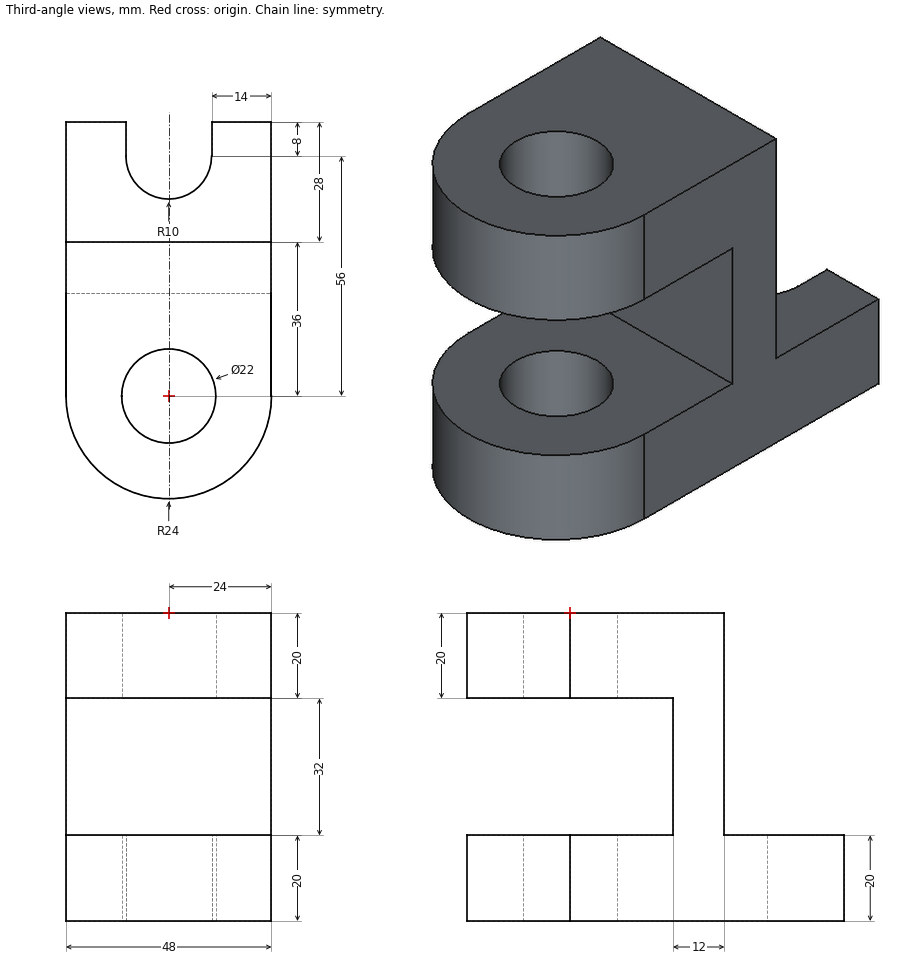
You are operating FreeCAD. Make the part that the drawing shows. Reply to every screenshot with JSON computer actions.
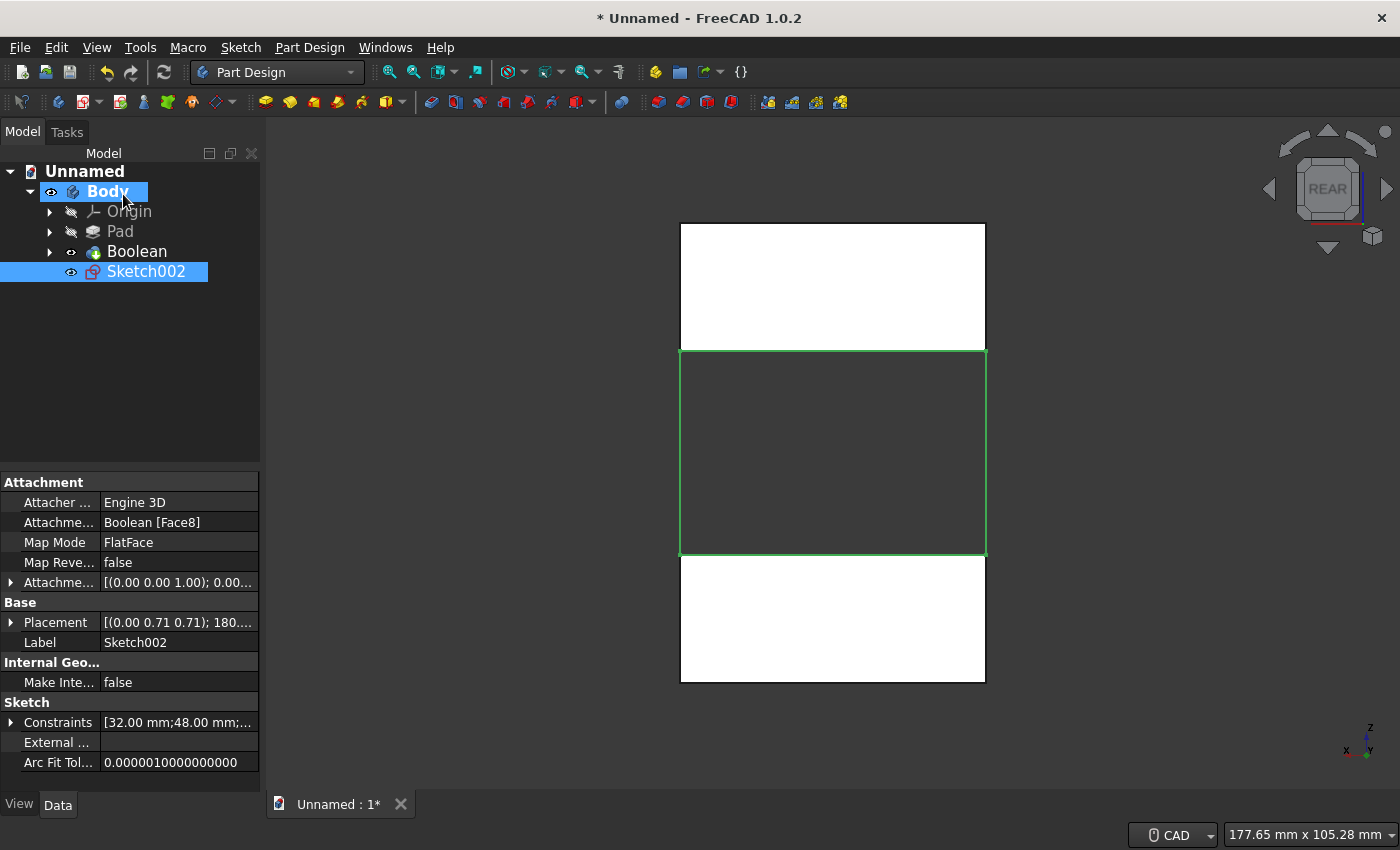
{"action": "left_click", "coordinate": [266, 102]}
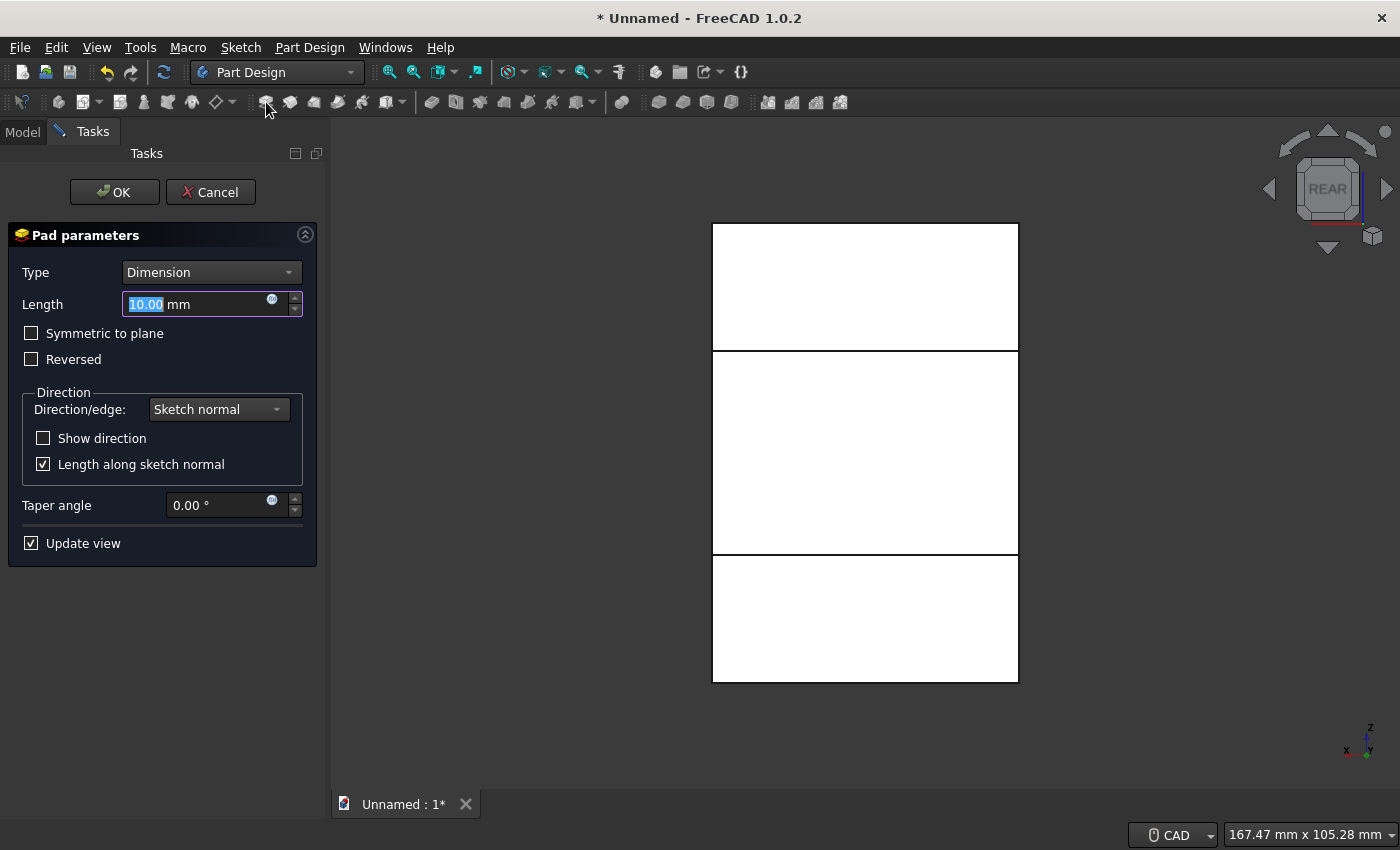
{"action": "type", "text": "12"}
{"action": "key", "text": "Tab"}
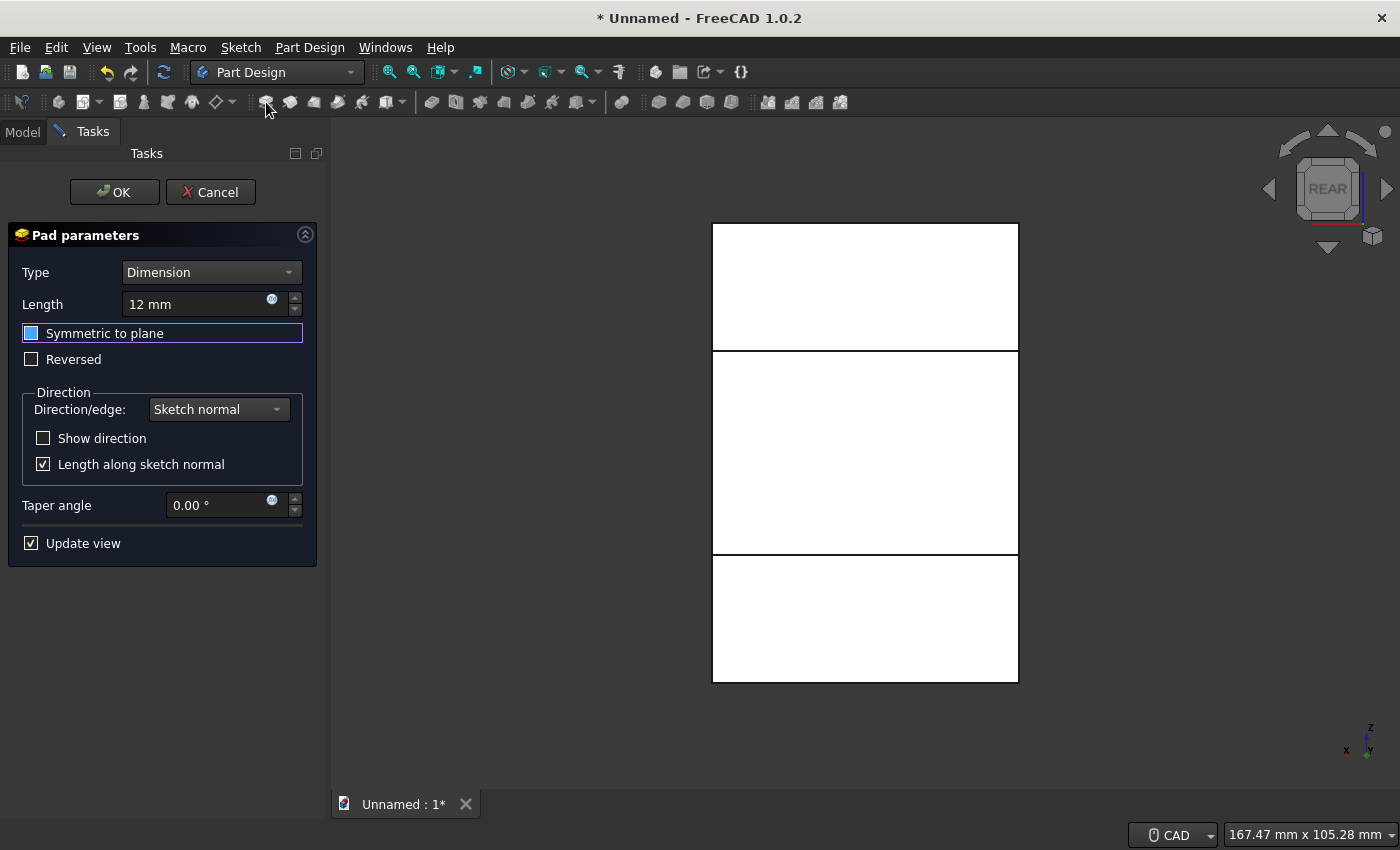
{"action": "left_click", "coordinate": [30, 359]}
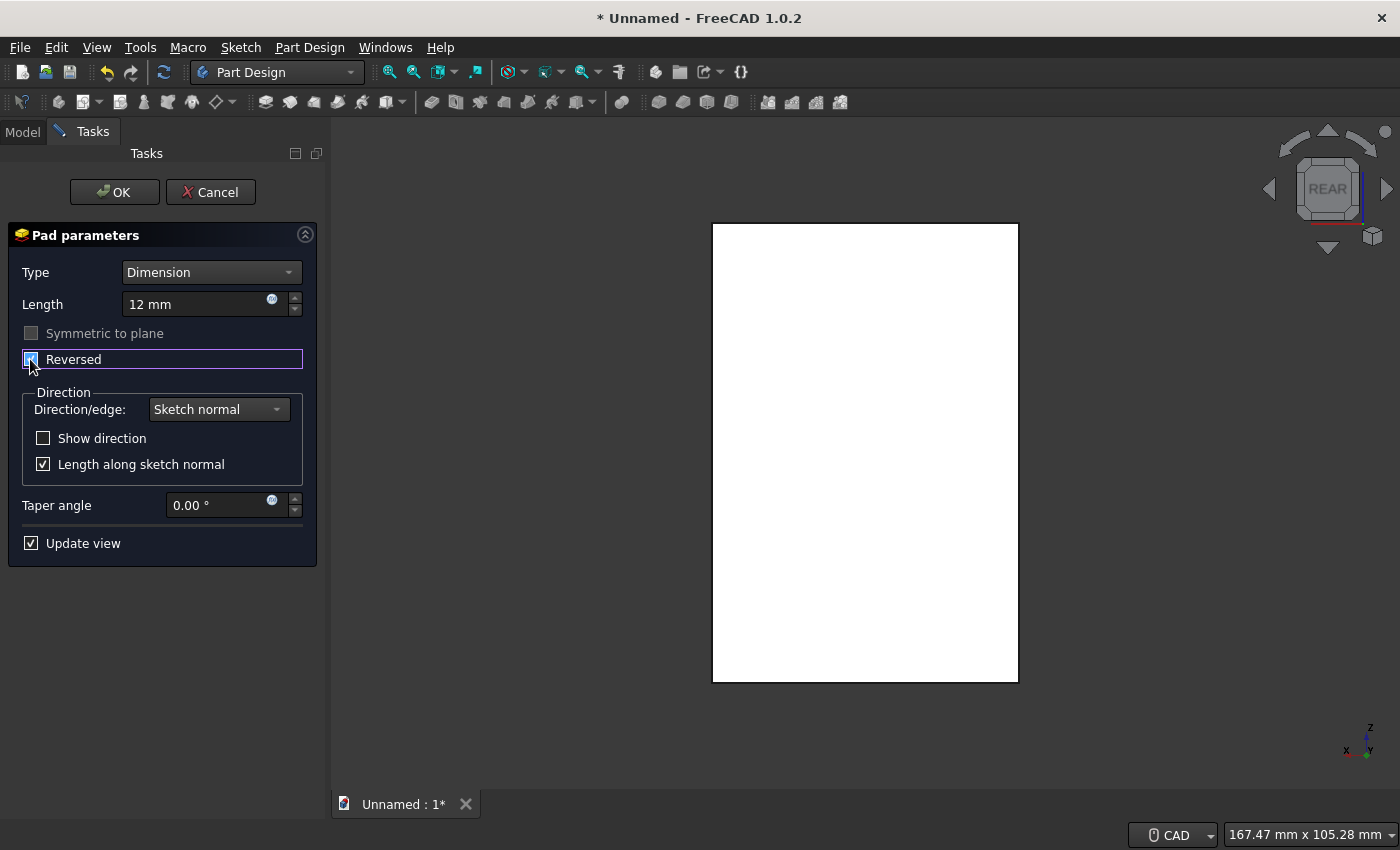
{"action": "left_click", "coordinate": [115, 192]}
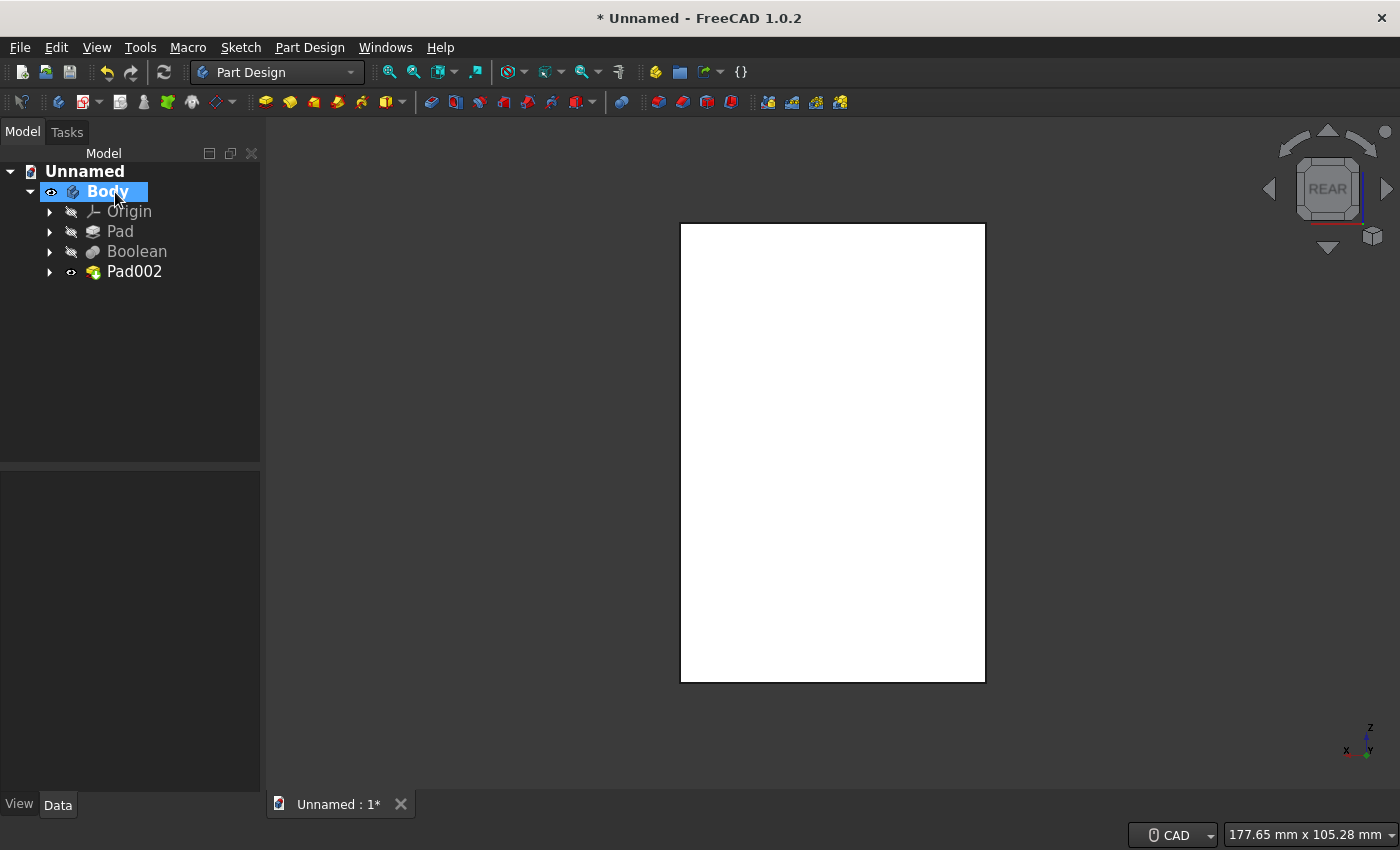
{"action": "key", "text": "5"}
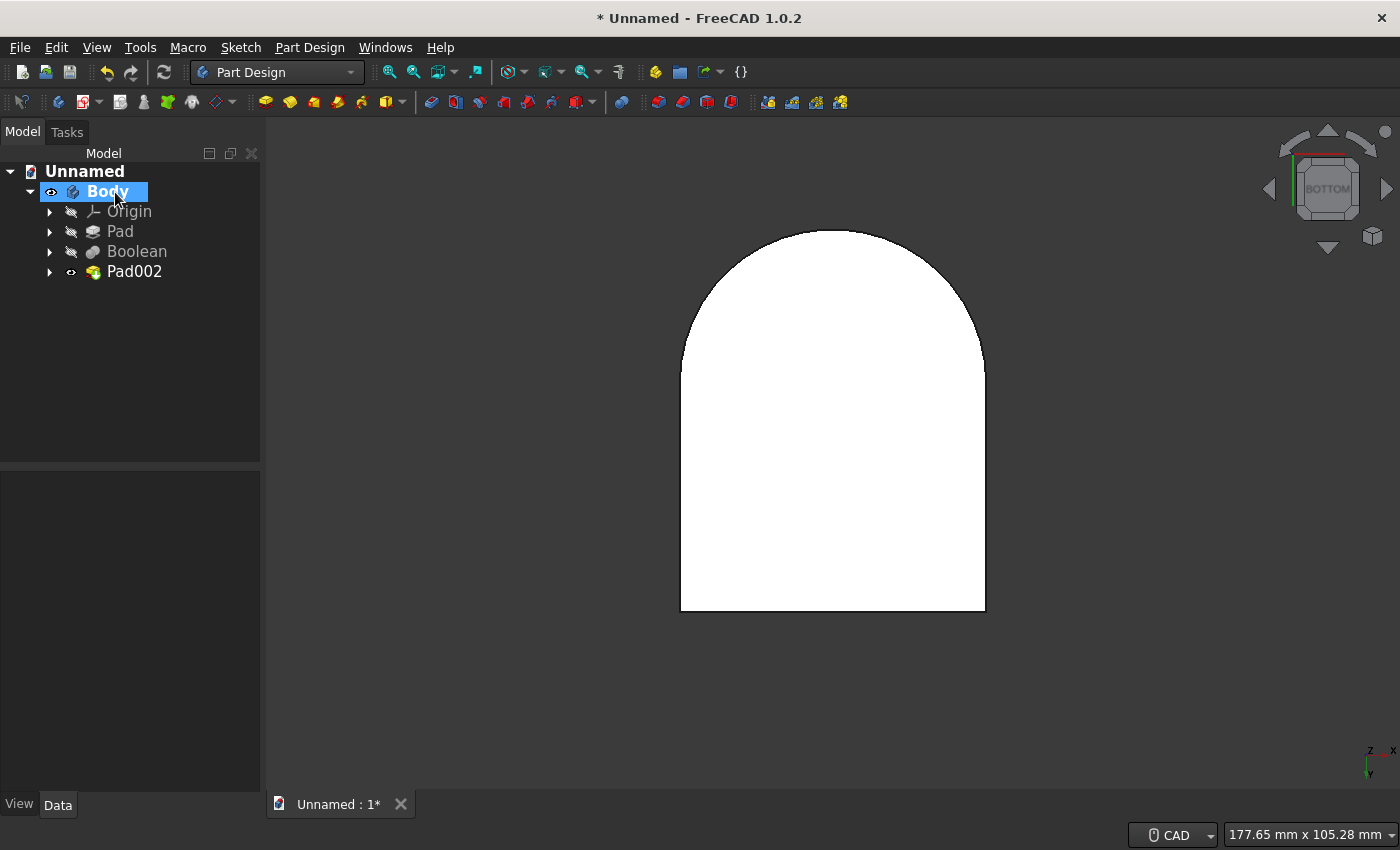
{"action": "left_click", "coordinate": [833, 420]}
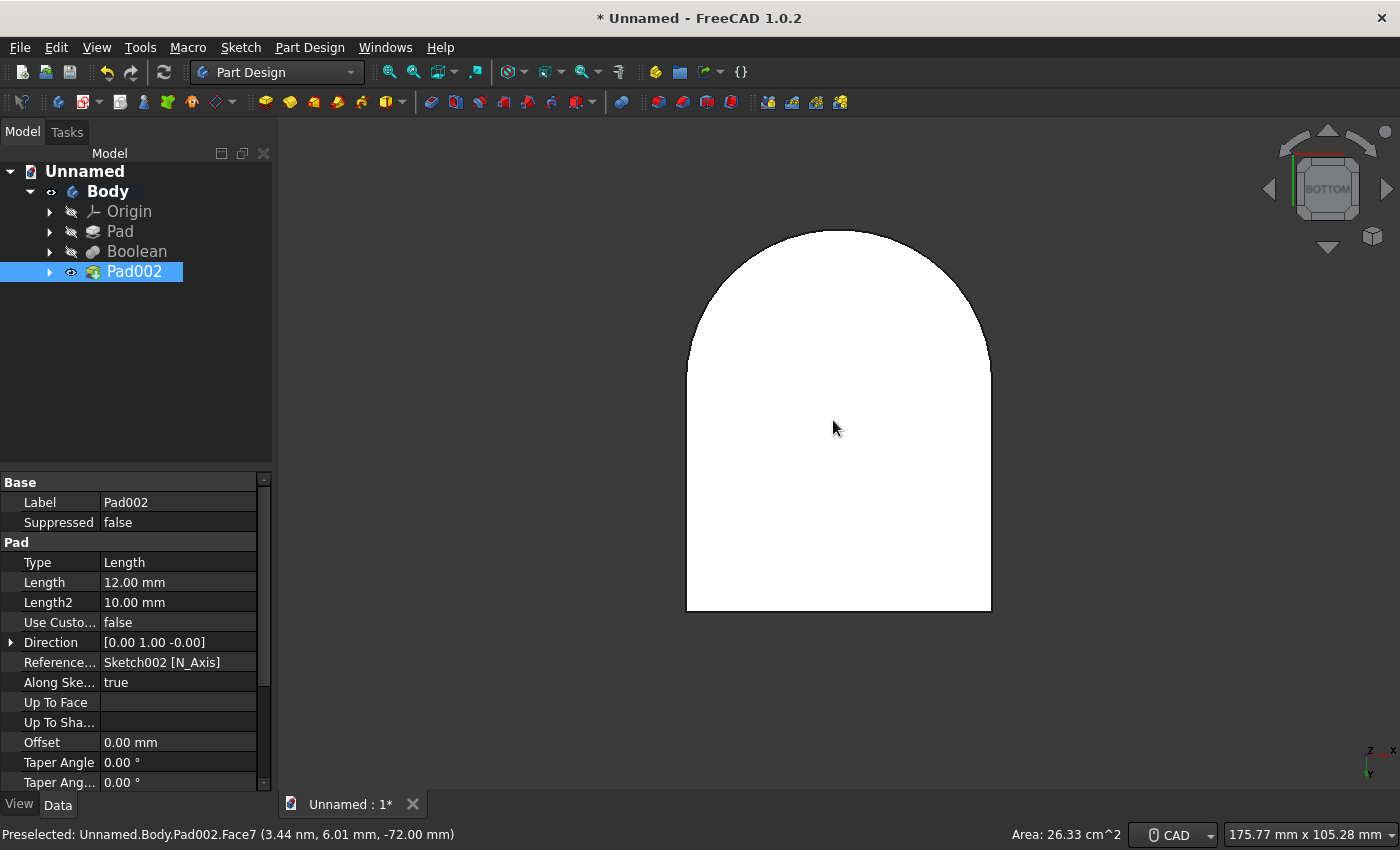
{"action": "left_click", "coordinate": [84, 102]}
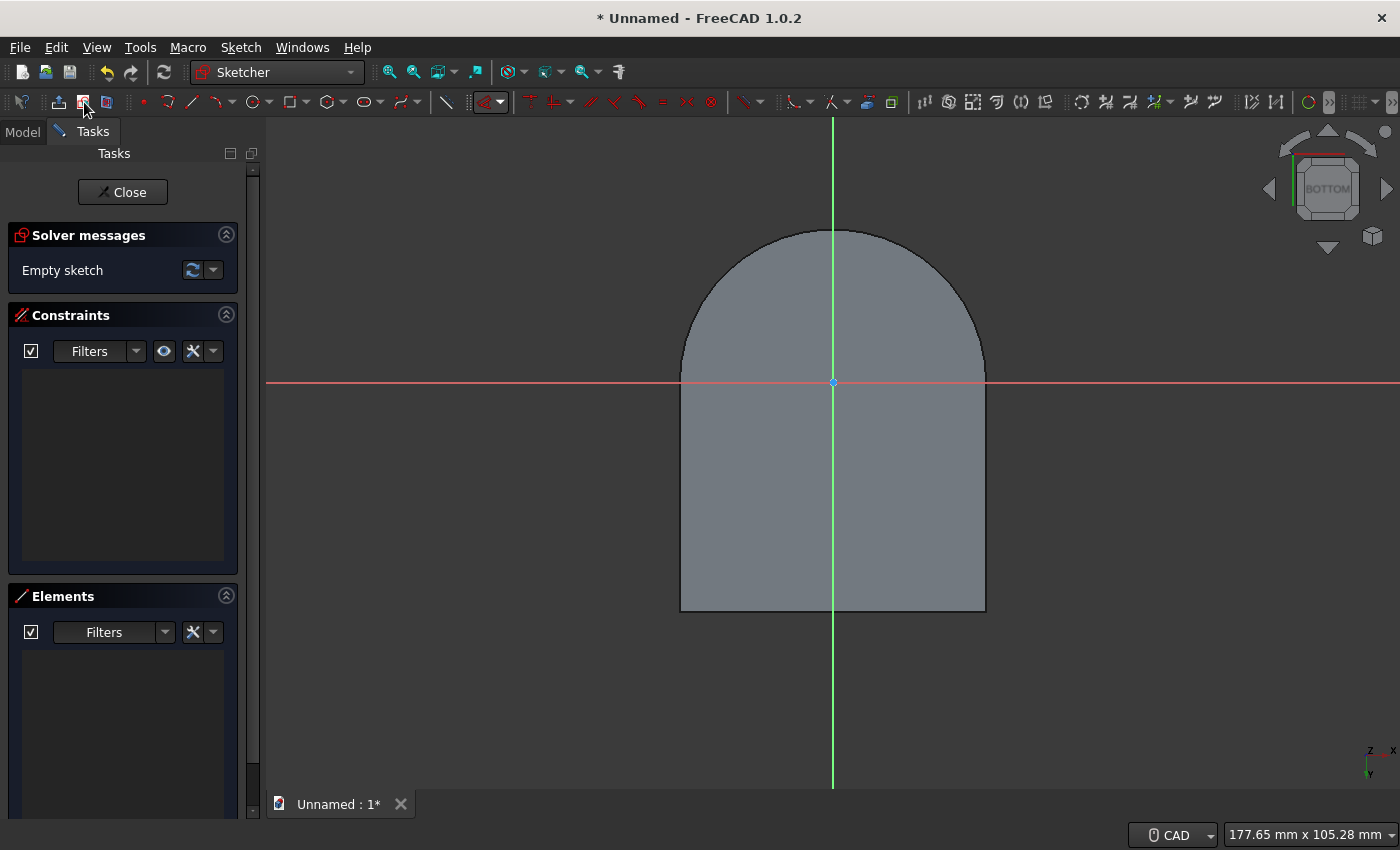
{"action": "scroll", "coordinate": [455, 145], "scroll_direction": "down", "scroll_amount": 1}